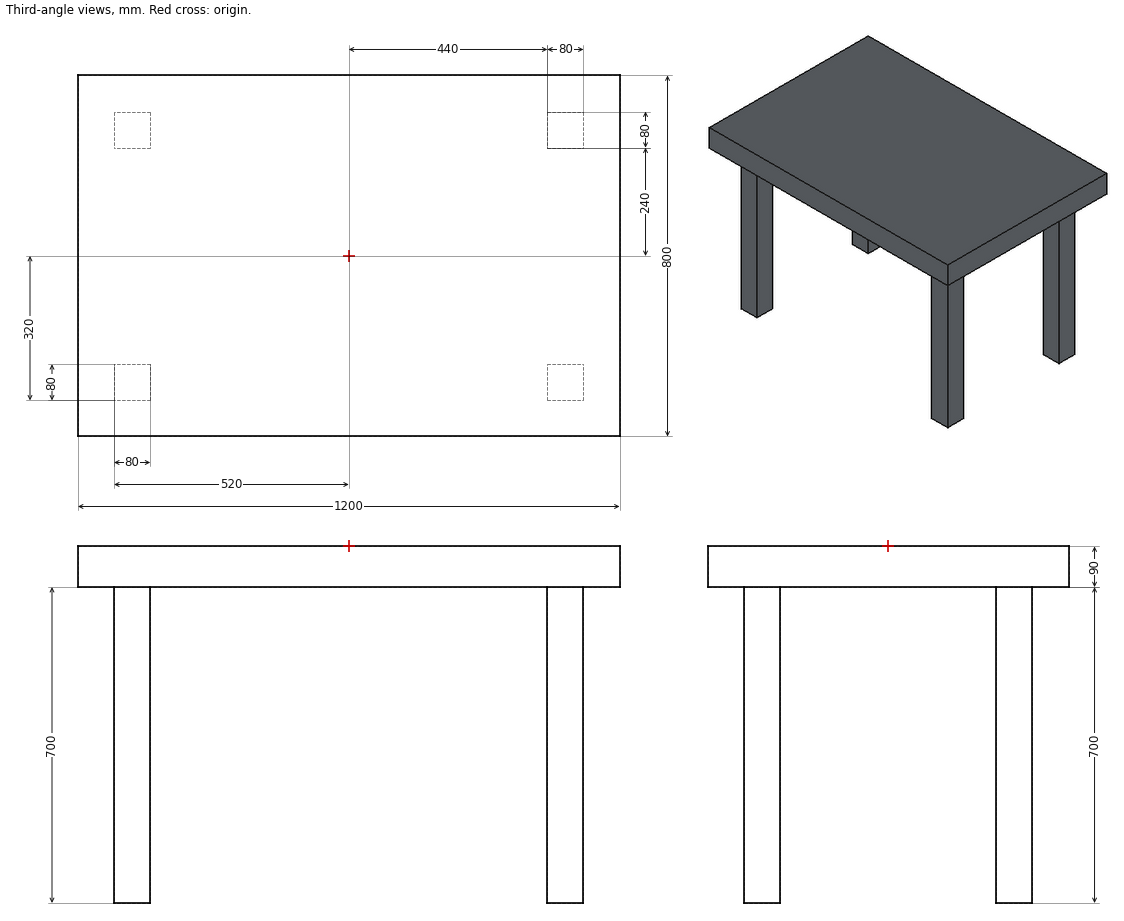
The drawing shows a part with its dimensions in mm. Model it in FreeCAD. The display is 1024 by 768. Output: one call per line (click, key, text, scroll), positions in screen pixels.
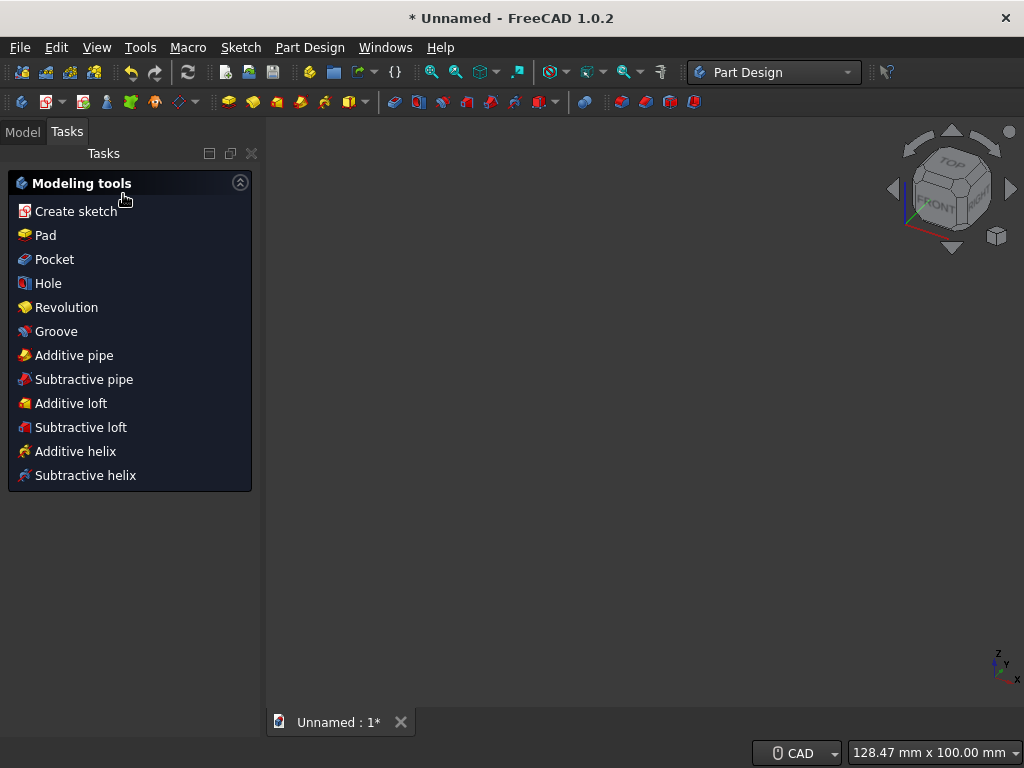
click(230, 102)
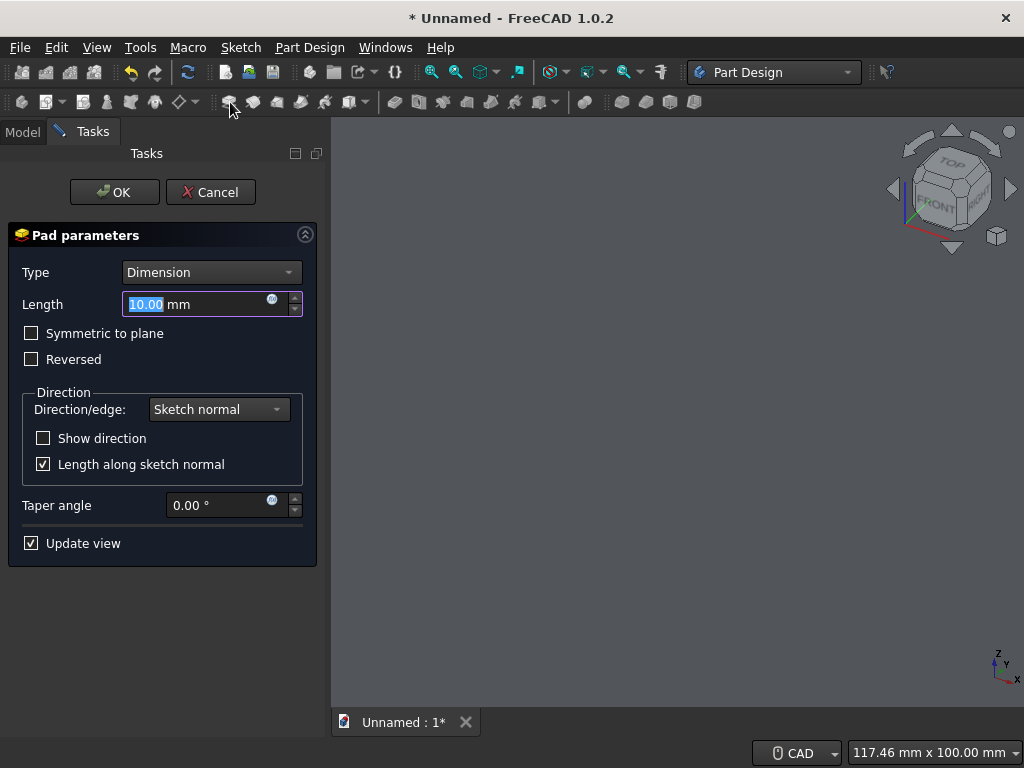
text(90)
key(Tab)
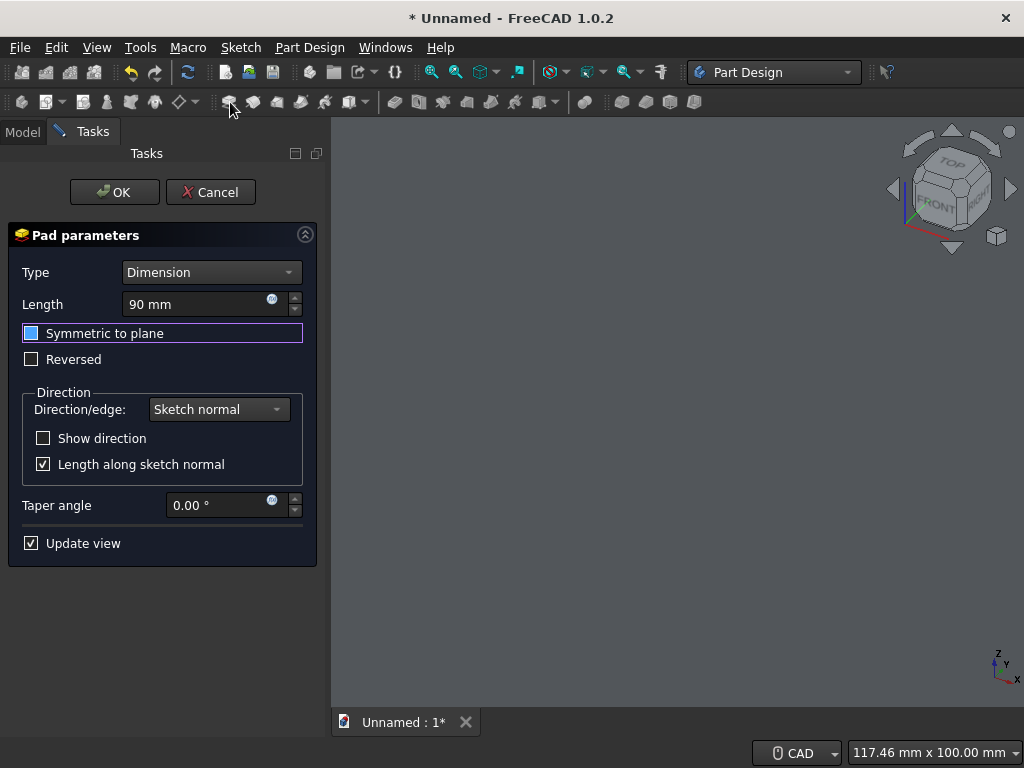
click(30, 359)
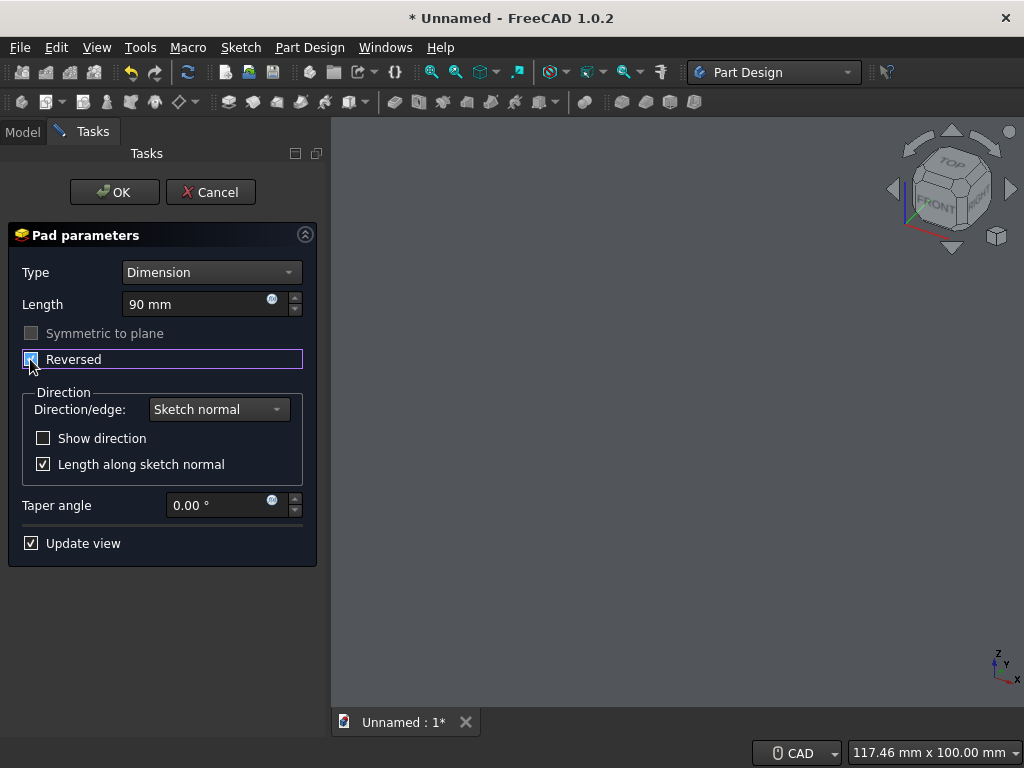
click(115, 192)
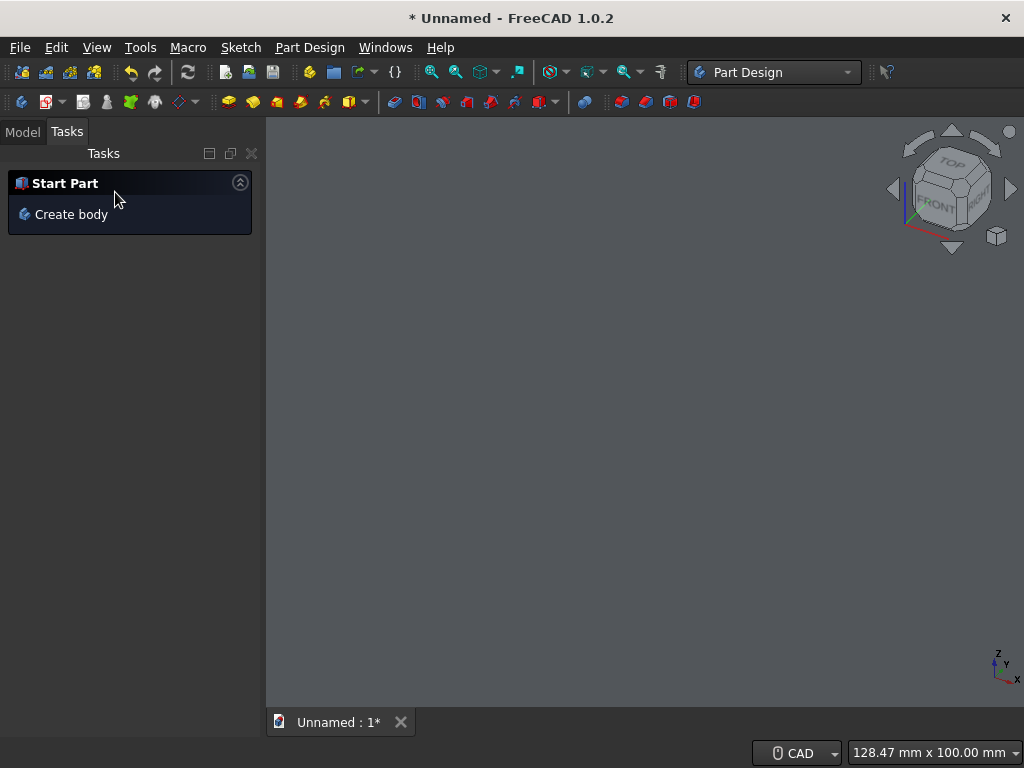
click(432, 72)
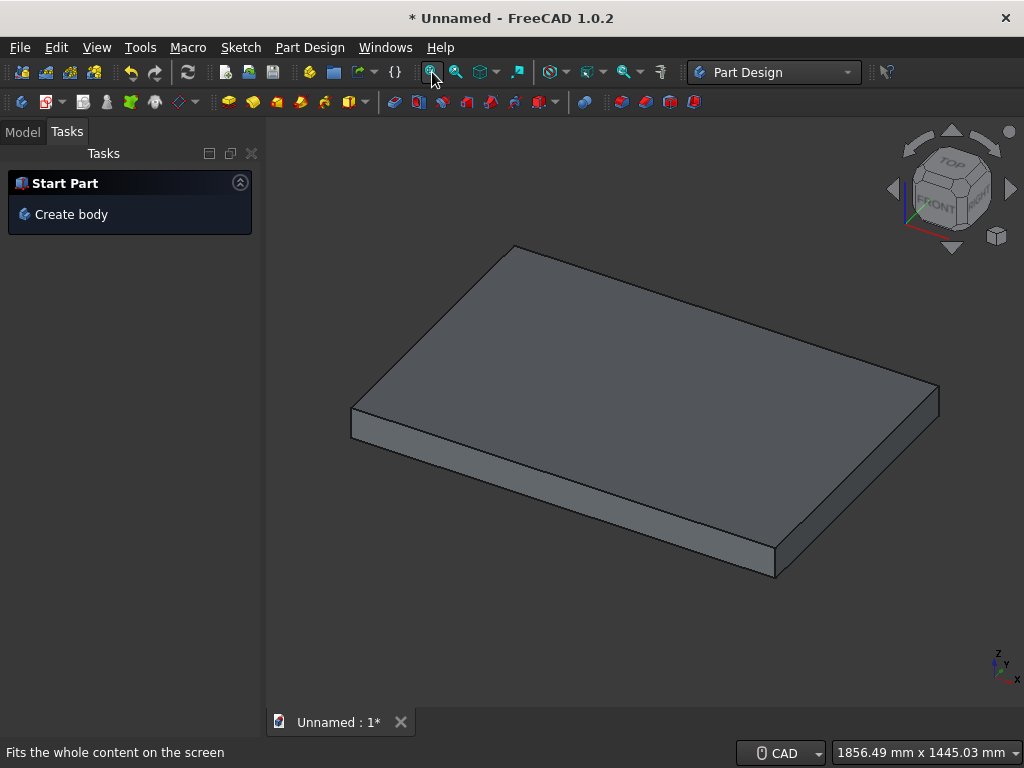
key(5)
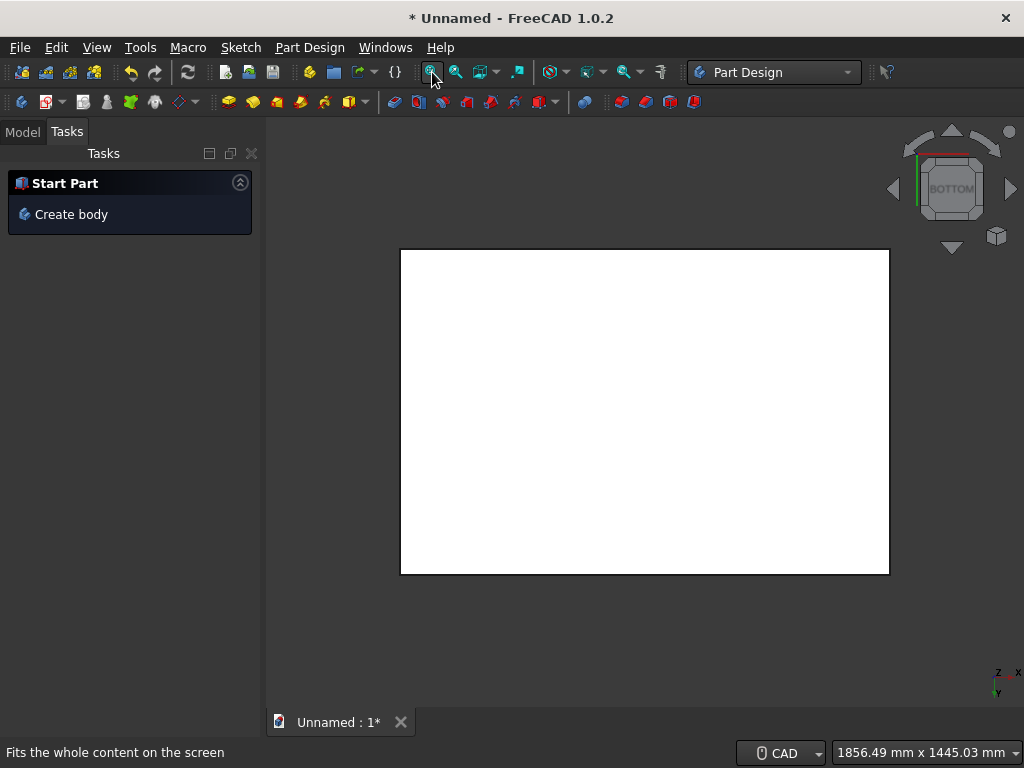
click(715, 411)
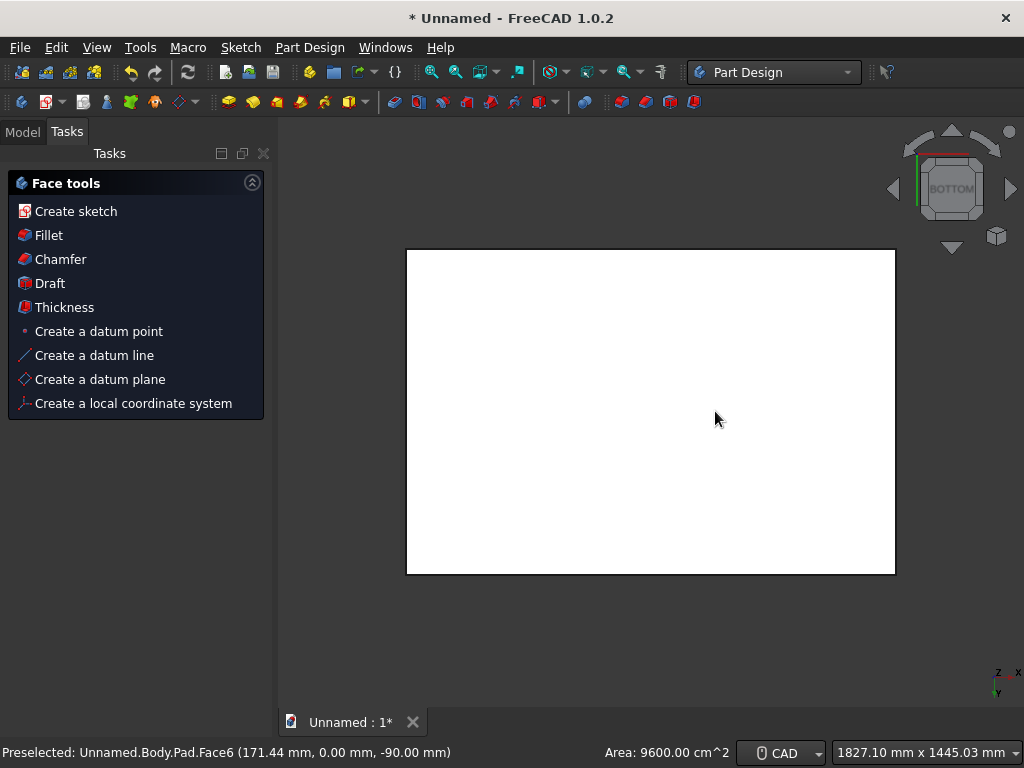
click(46, 102)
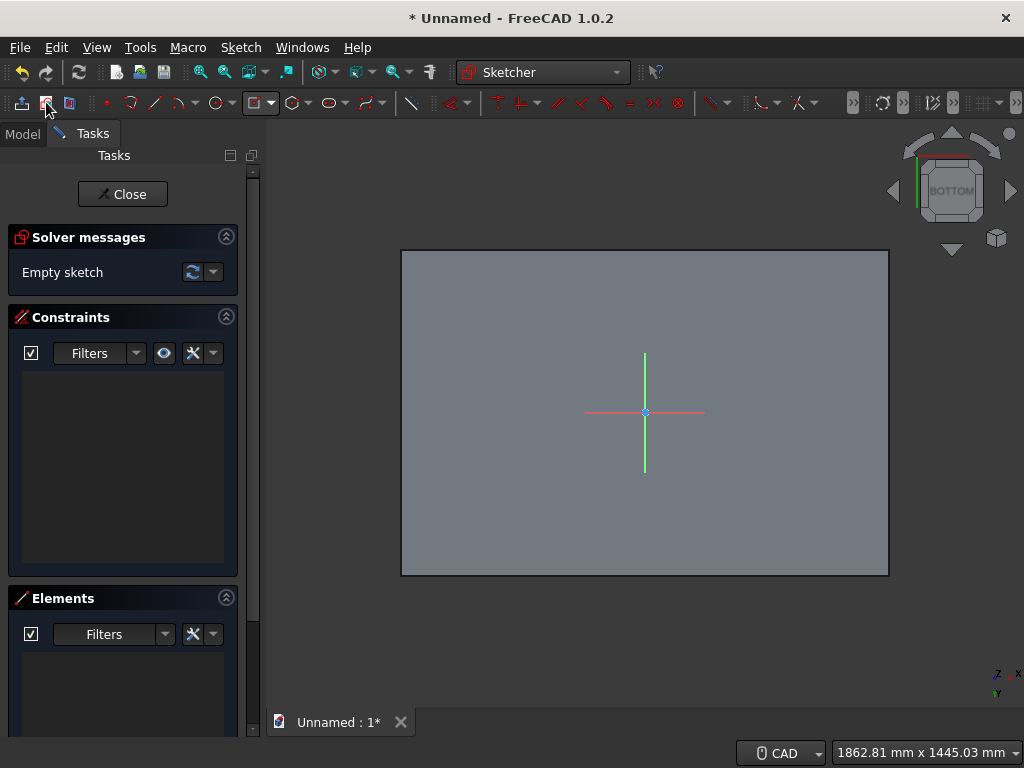
scroll(437, 288, up, 12)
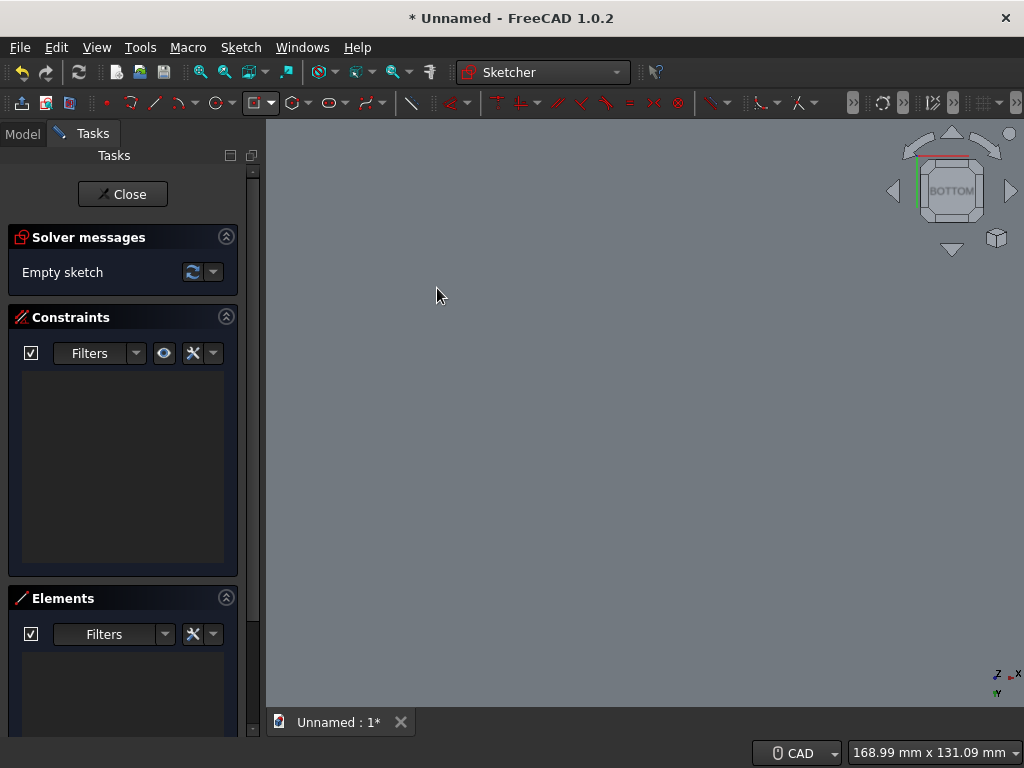
click(274, 104)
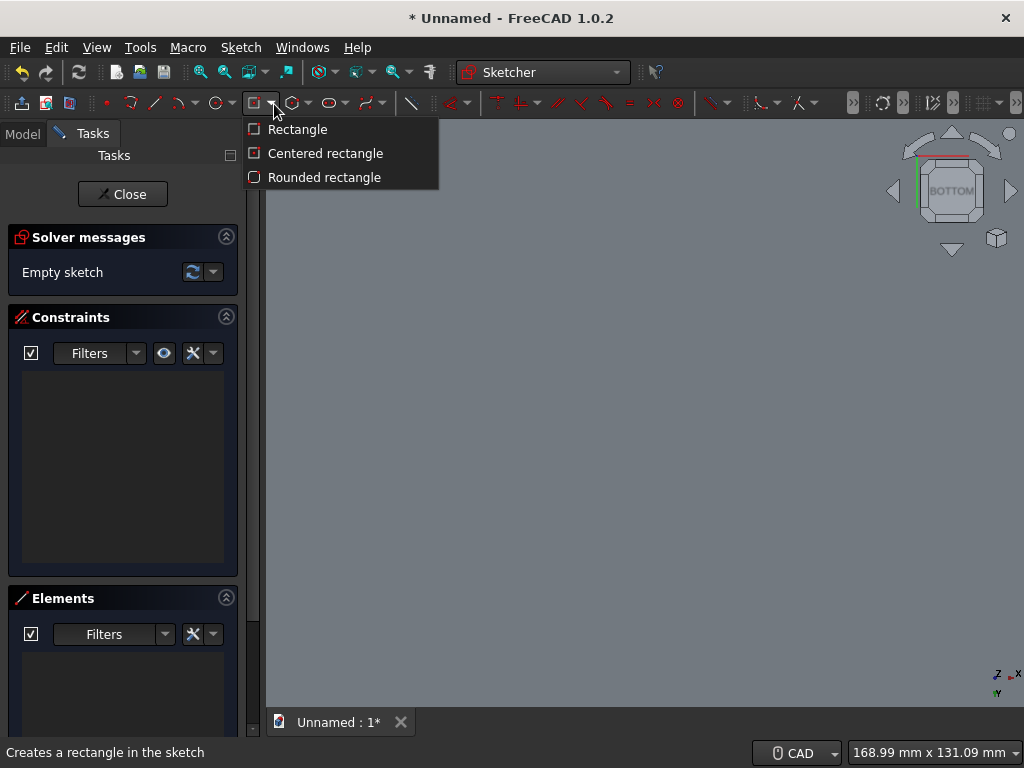
click(340, 129)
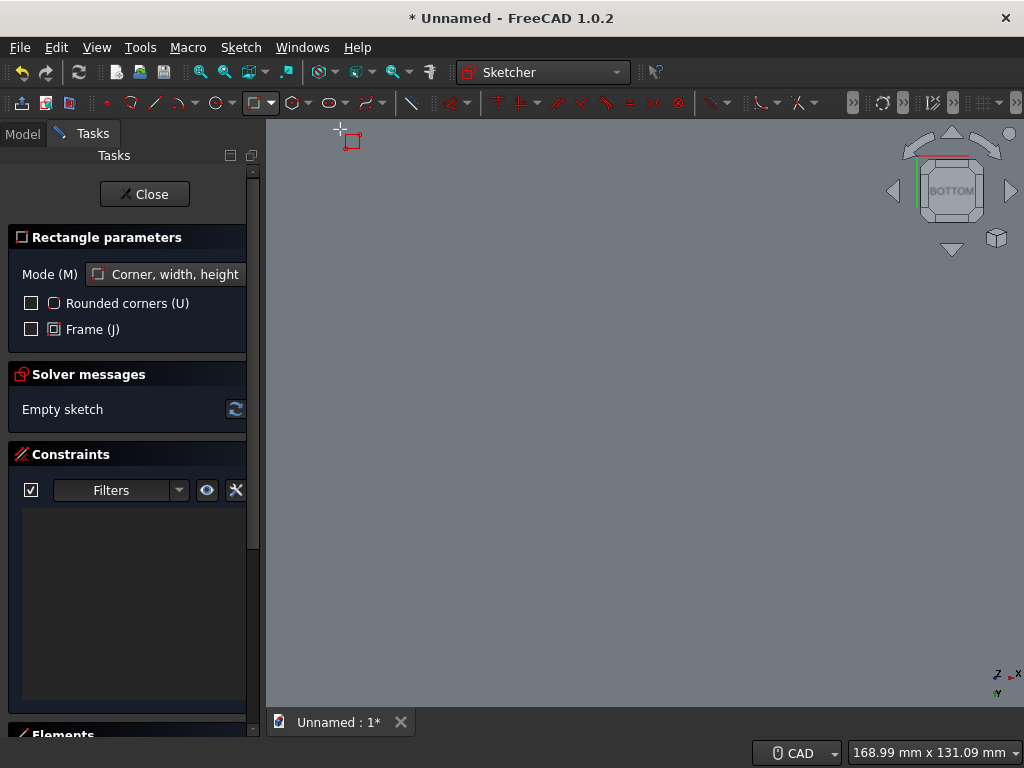
click(395, 228)
click(754, 586)
key(Escape)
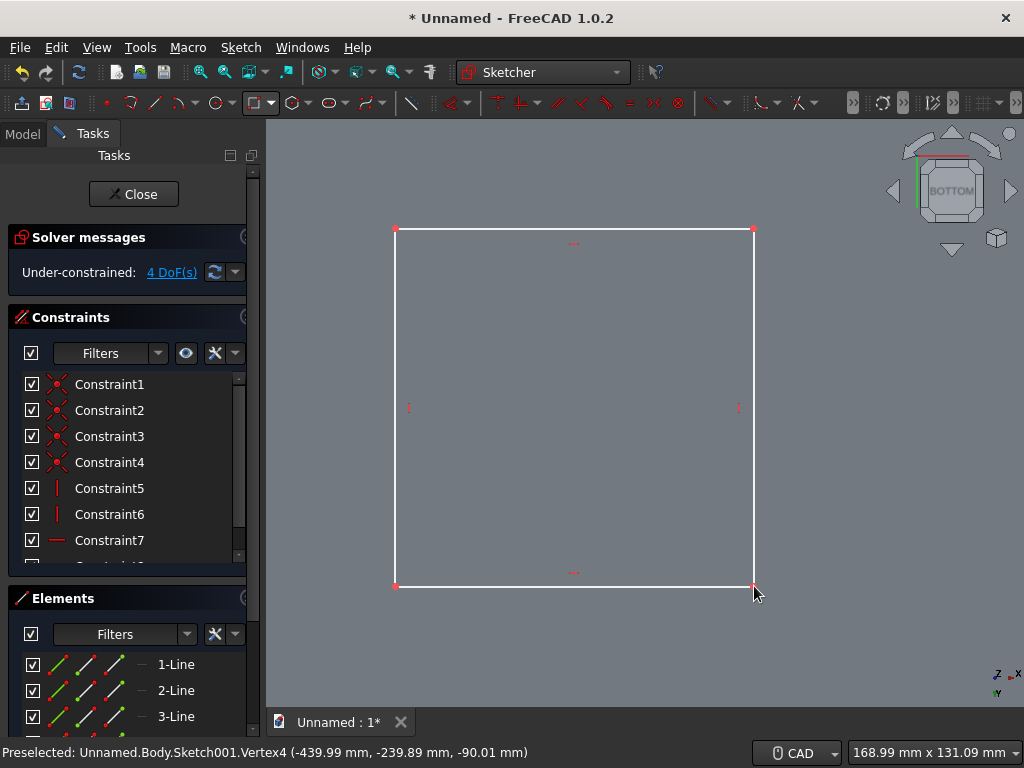
key(d)